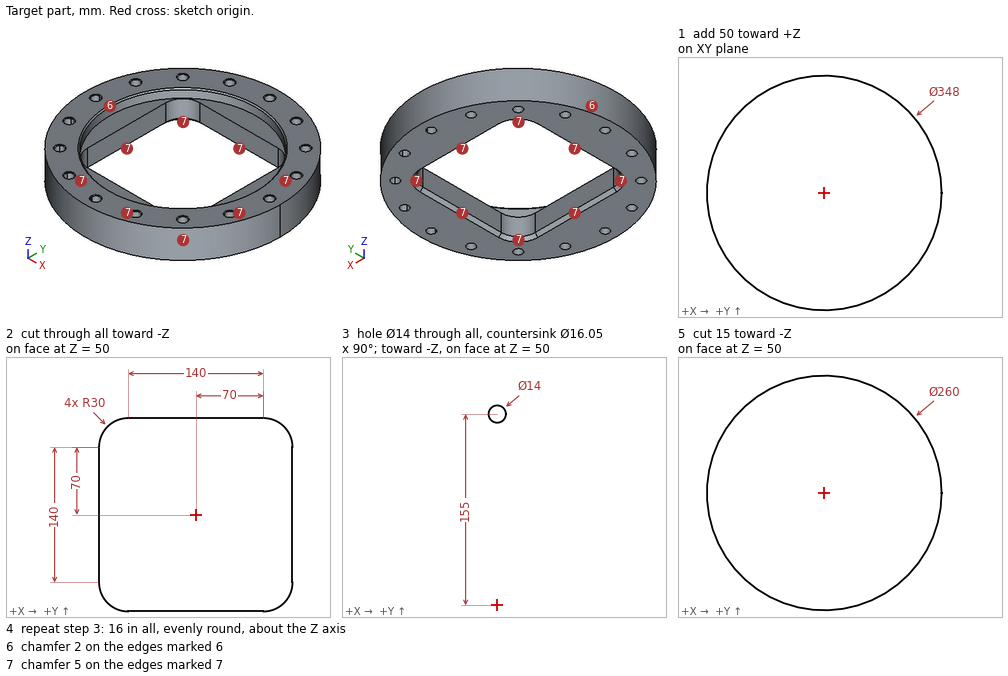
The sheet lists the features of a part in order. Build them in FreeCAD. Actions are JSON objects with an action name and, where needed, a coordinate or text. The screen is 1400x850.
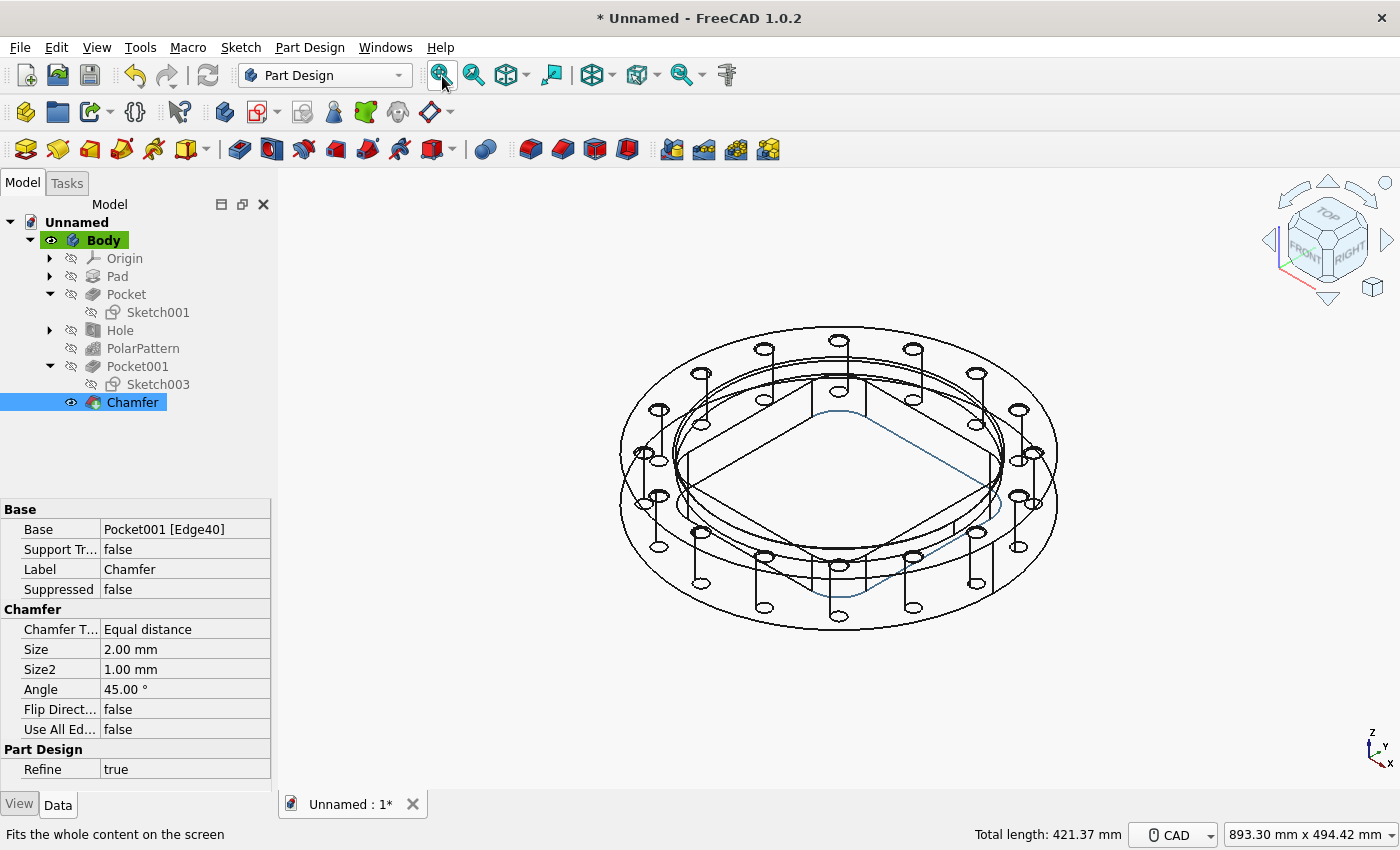
{"action": "left_click", "coordinate": [677, 503], "text": "ctrl"}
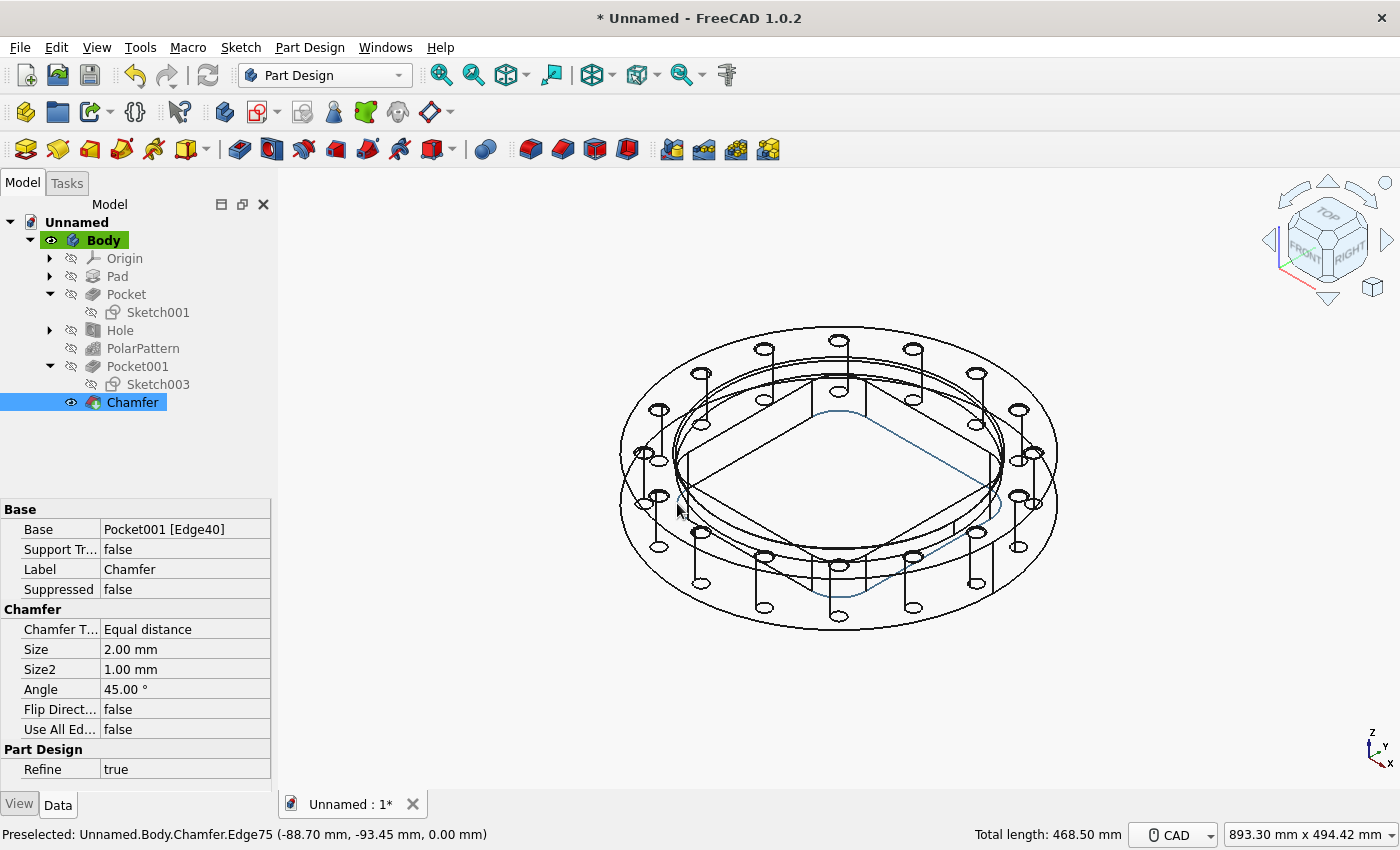
{"action": "left_click", "coordinate": [750, 452], "text": "ctrl"}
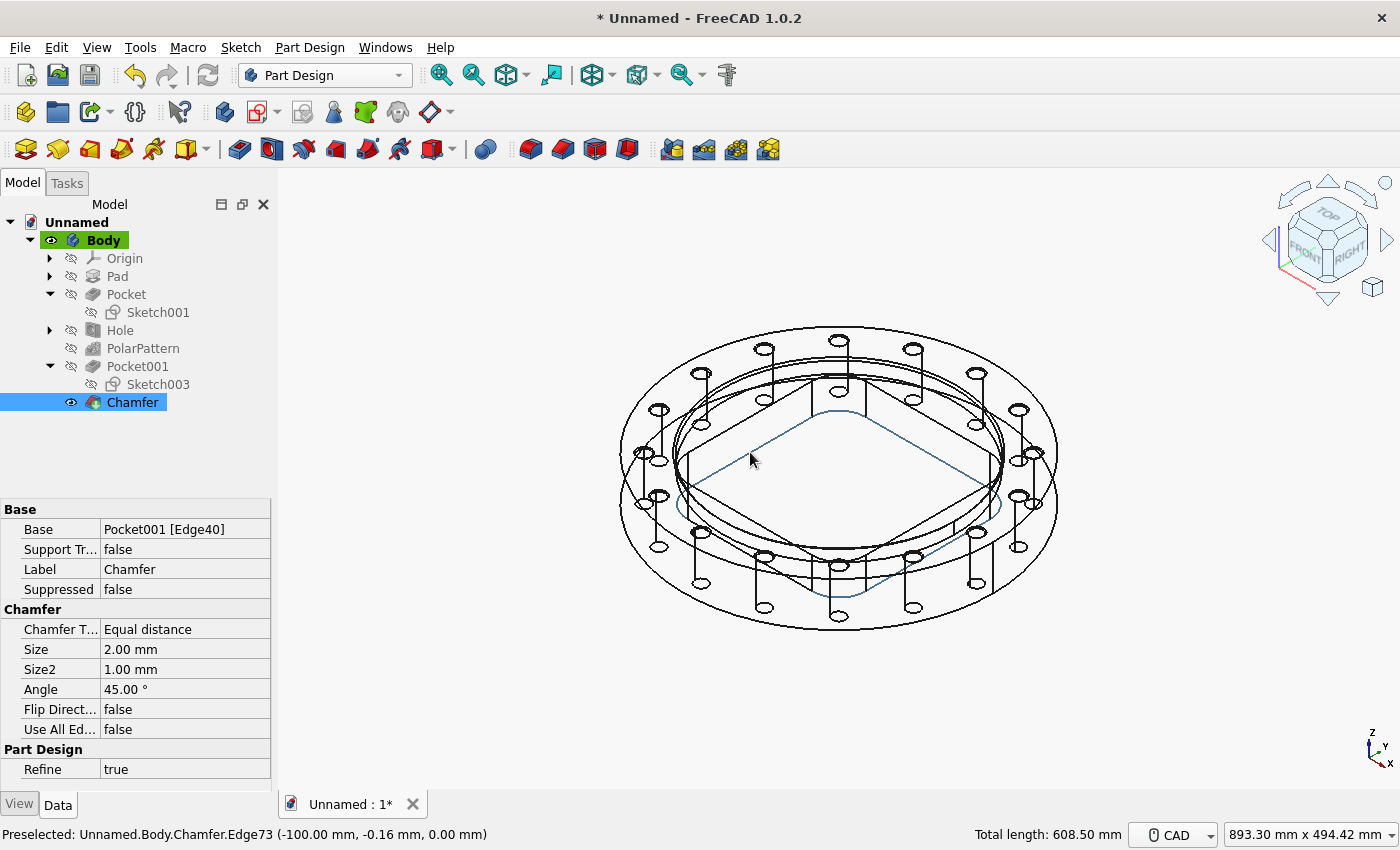
{"action": "left_click", "coordinate": [797, 582], "text": "ctrl"}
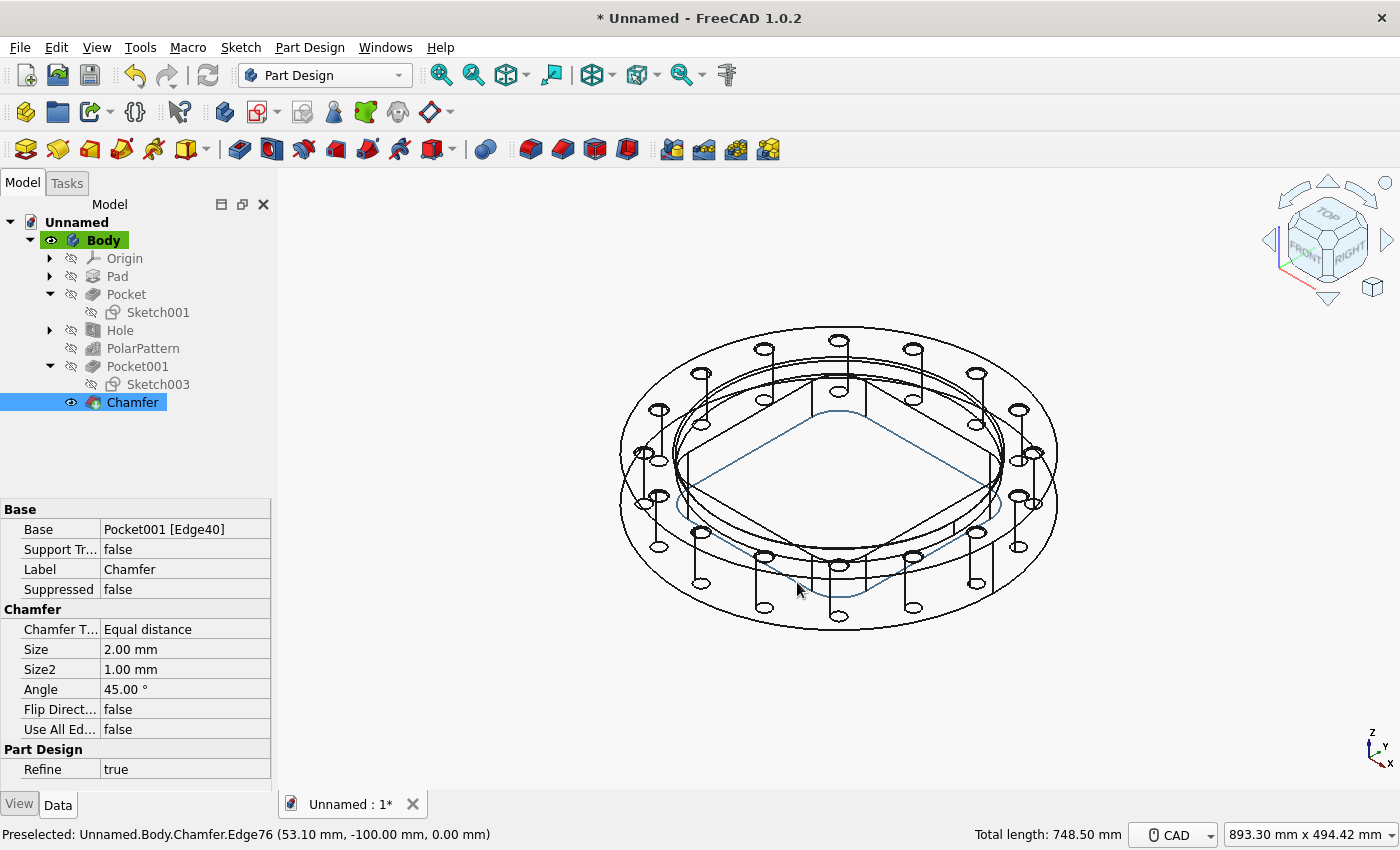
{"action": "key", "text": "v 1"}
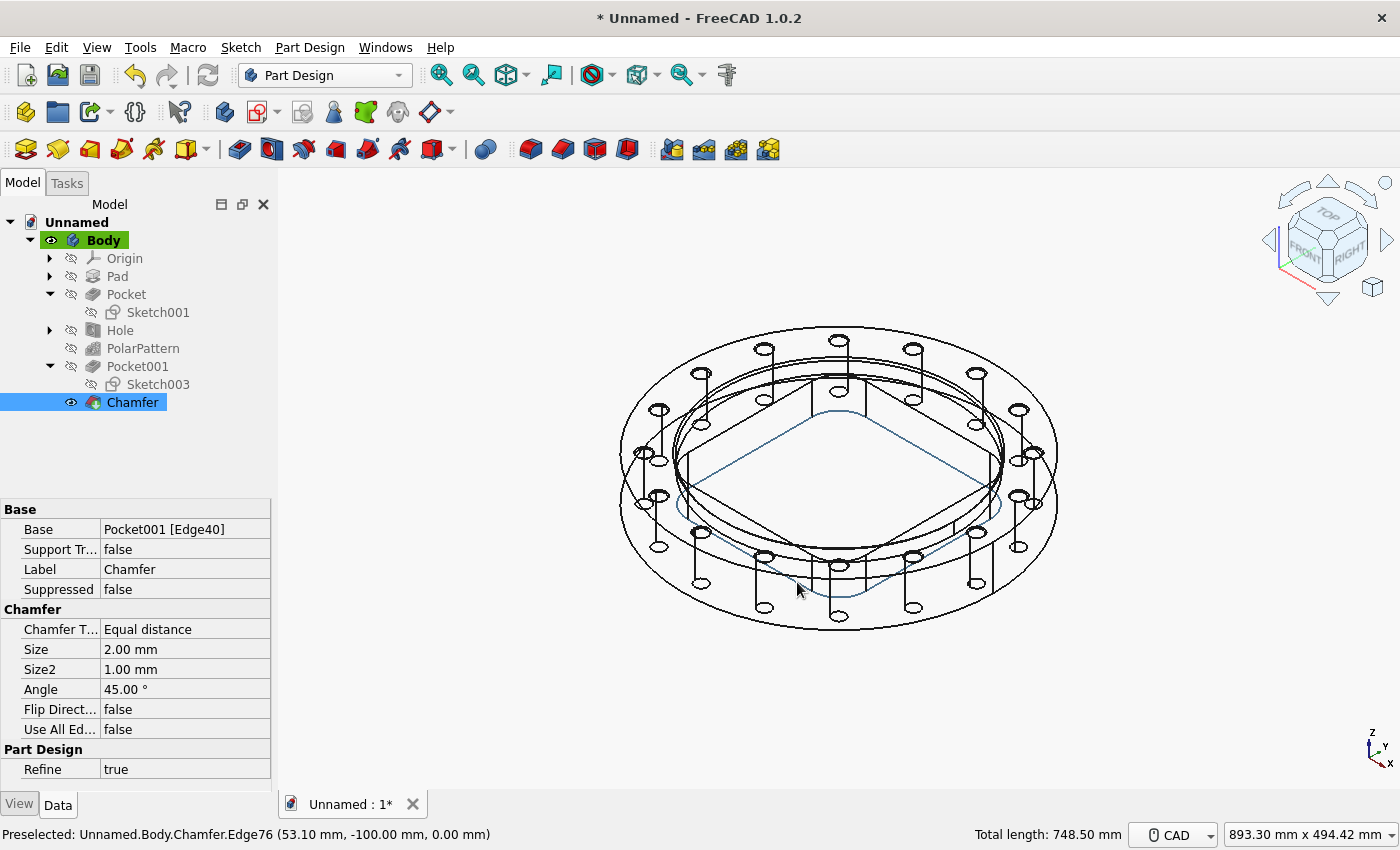
{"action": "left_click", "coordinate": [564, 150]}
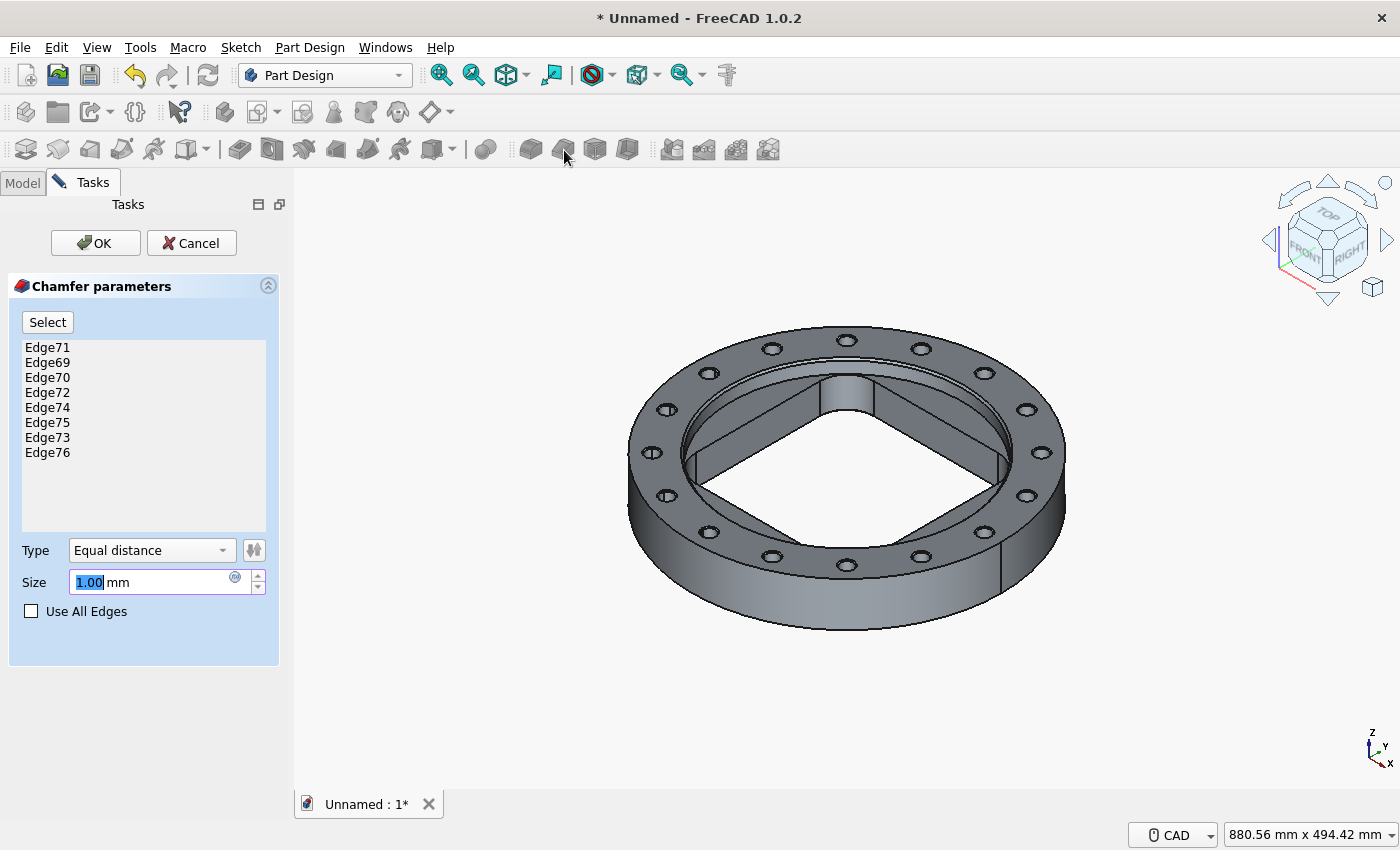
{"action": "type", "text": "5"}
{"action": "key", "text": "Tab"}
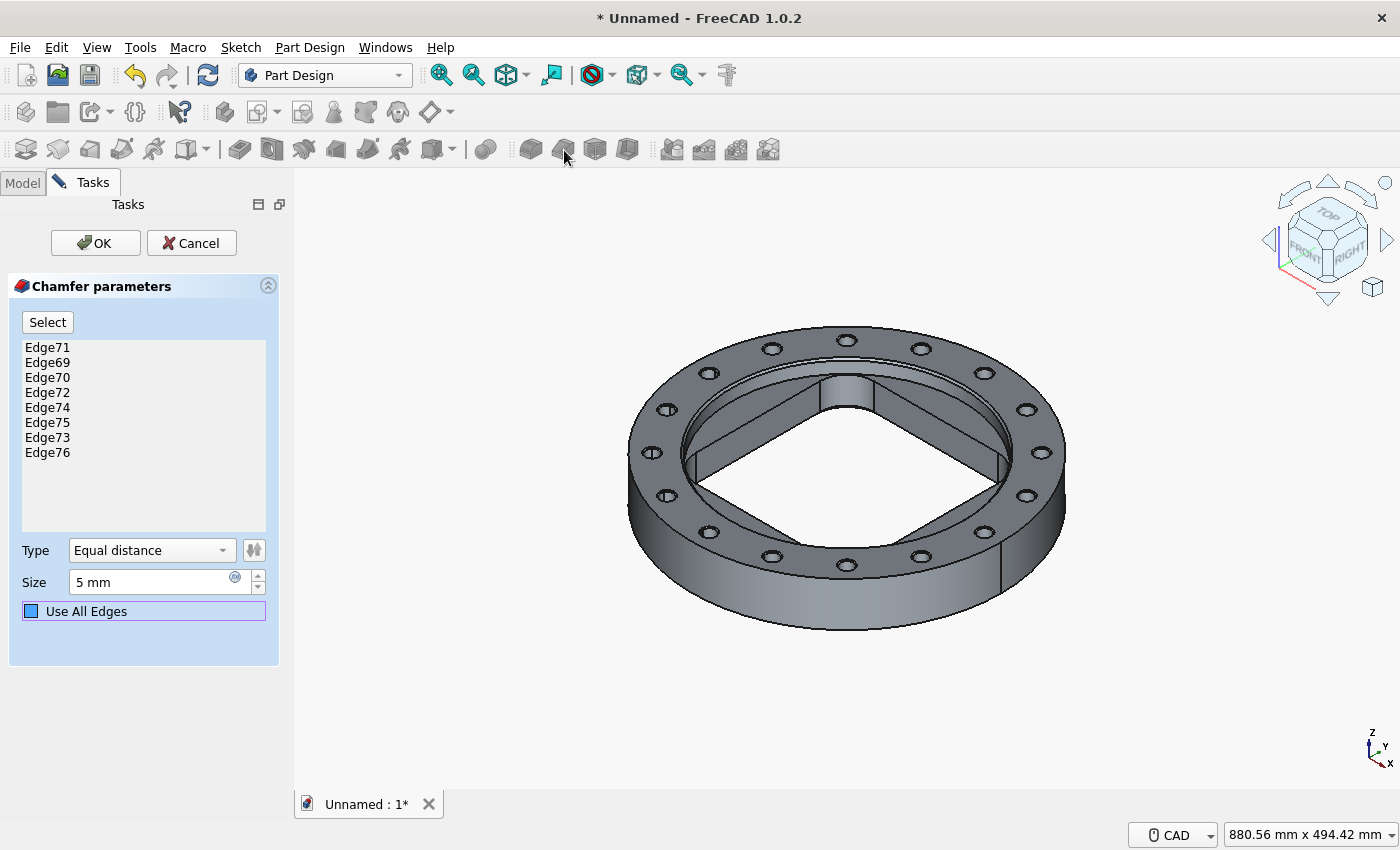
{"action": "left_click", "coordinate": [96, 243]}